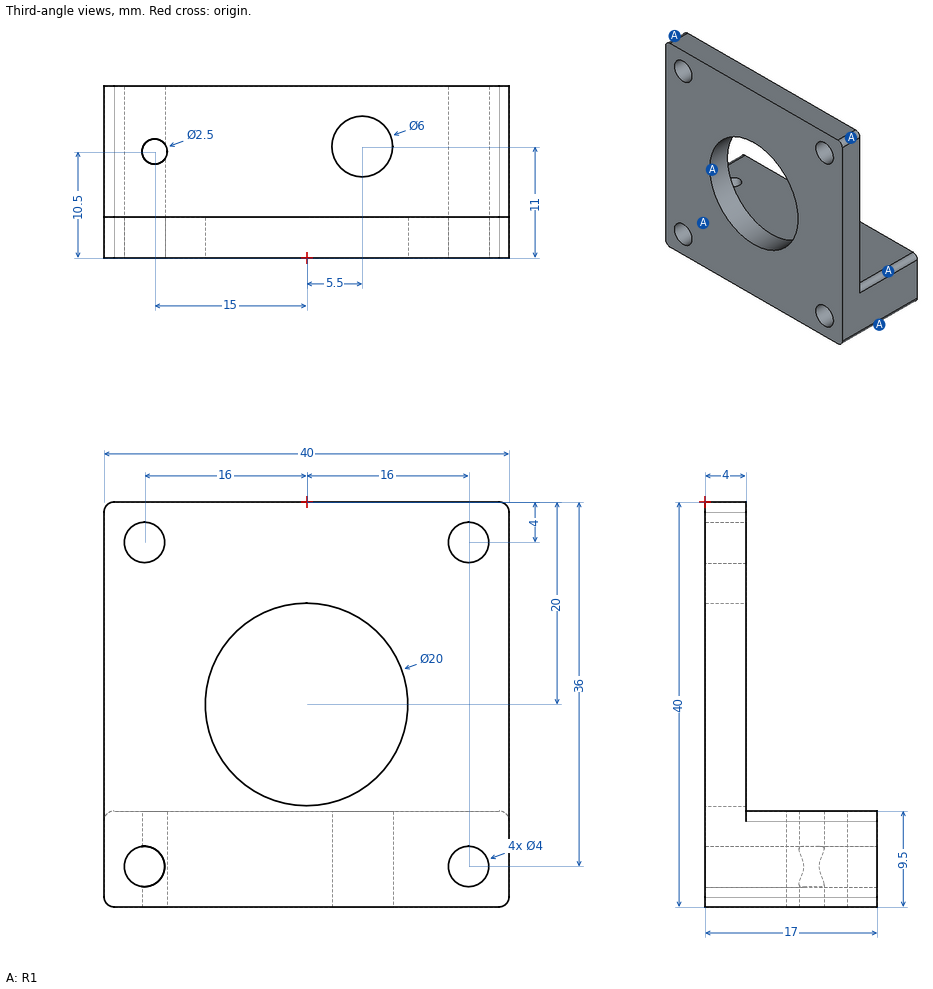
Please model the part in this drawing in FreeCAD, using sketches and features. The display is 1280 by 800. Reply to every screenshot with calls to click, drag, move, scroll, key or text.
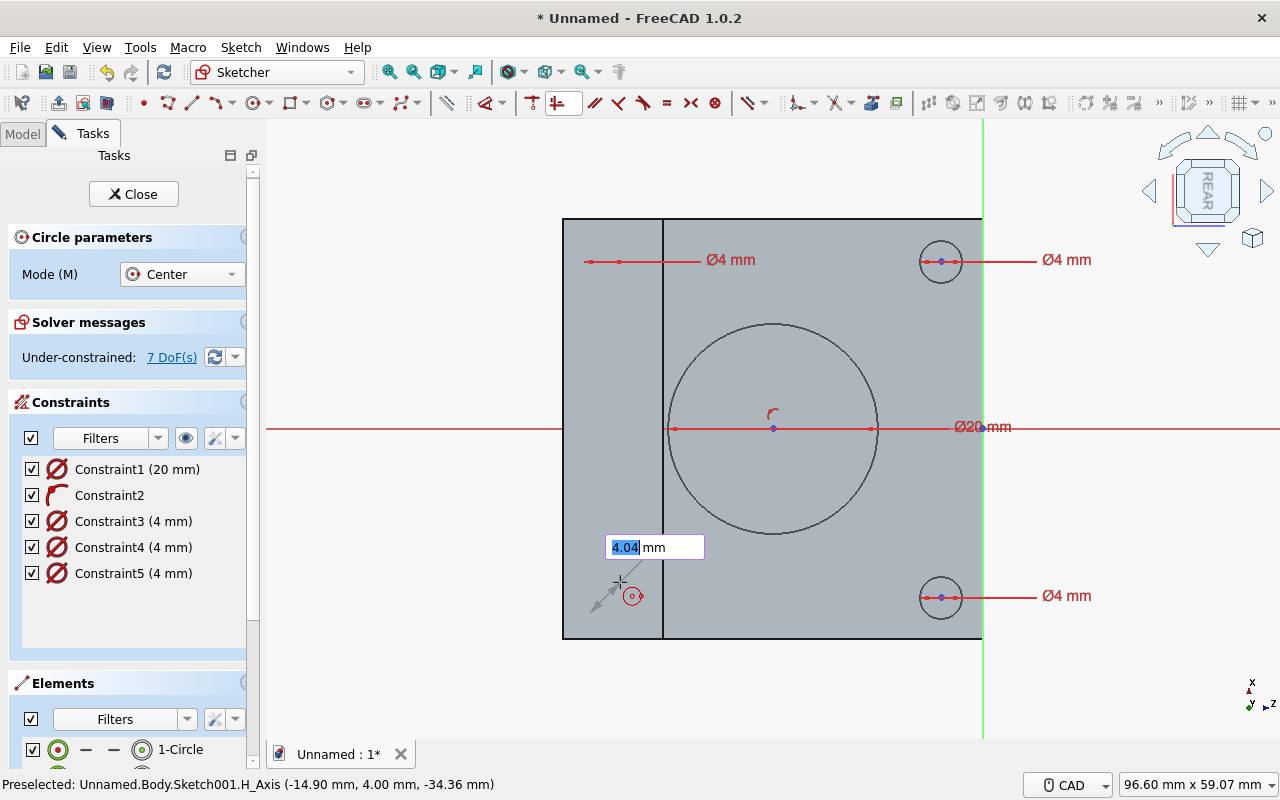
text(4)
key(Return)
key(Escape)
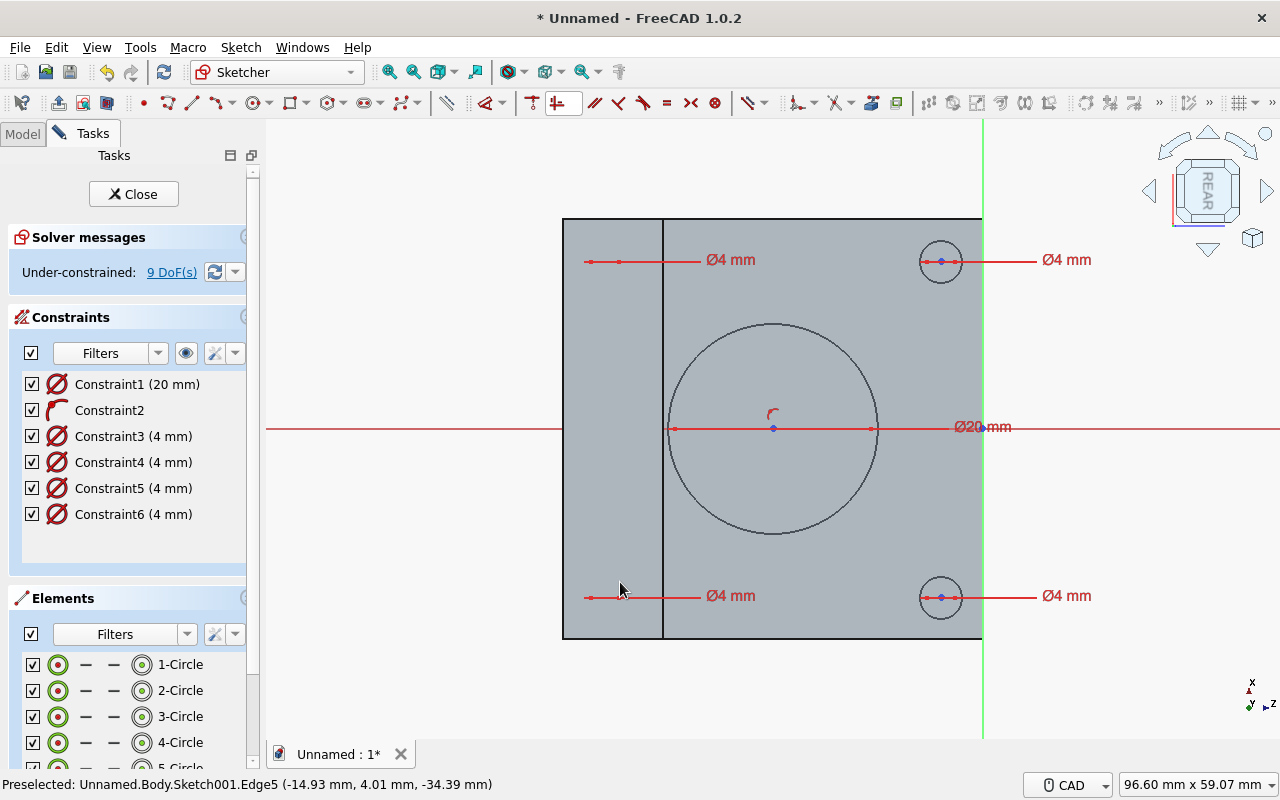
click(605, 262)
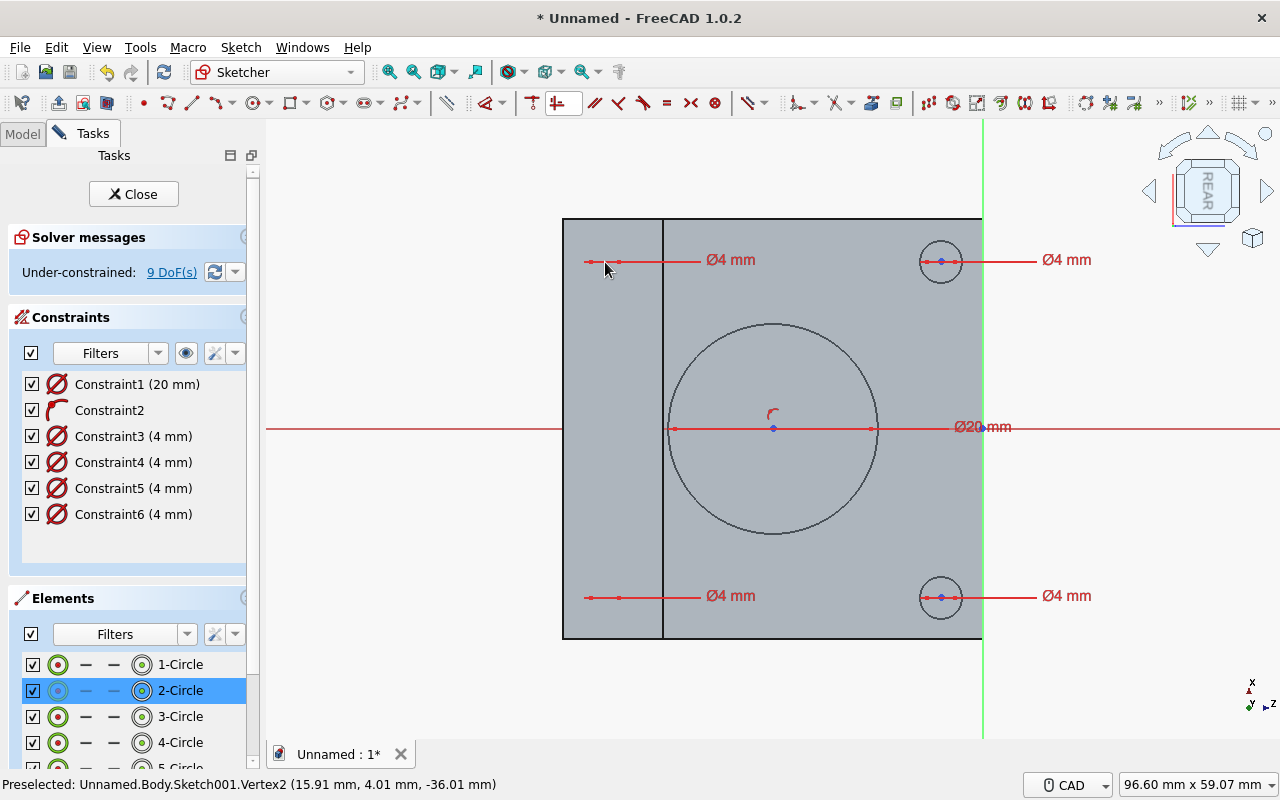
click(941, 262)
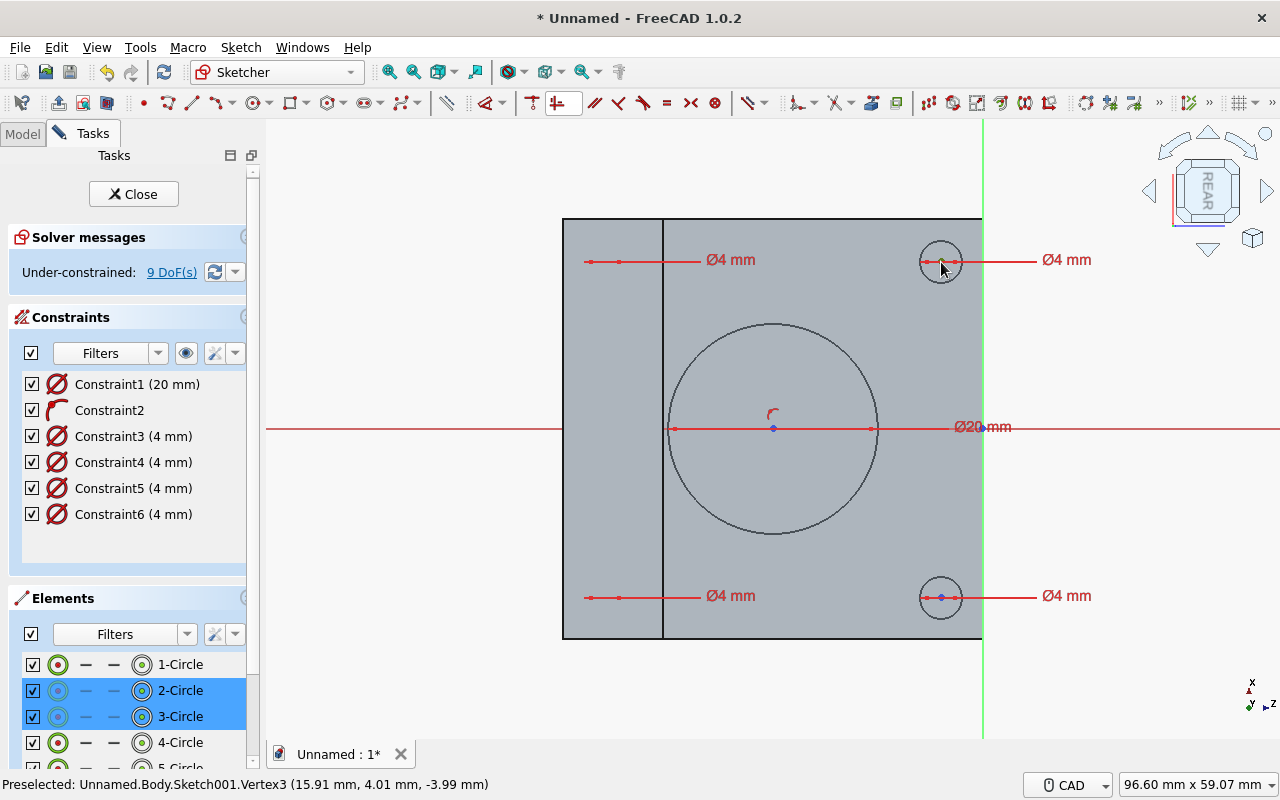
click(576, 104)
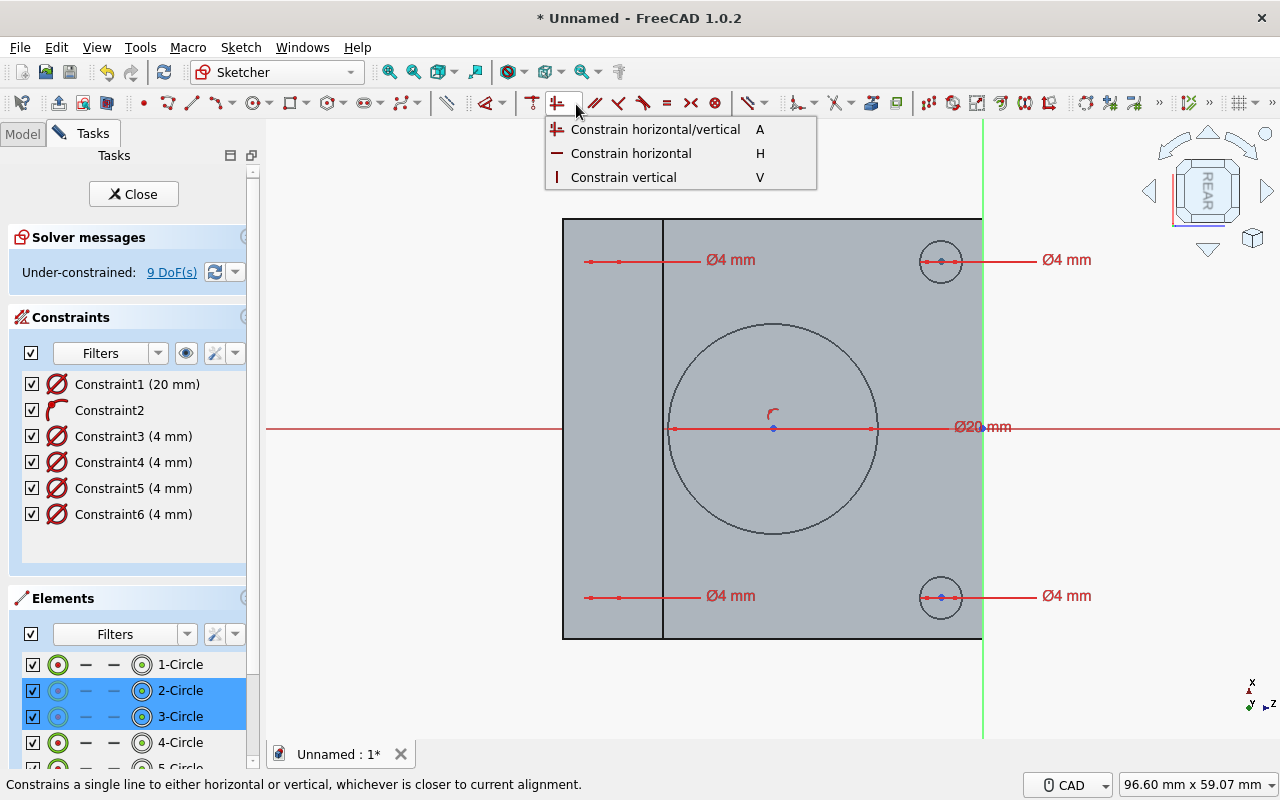
click(681, 153)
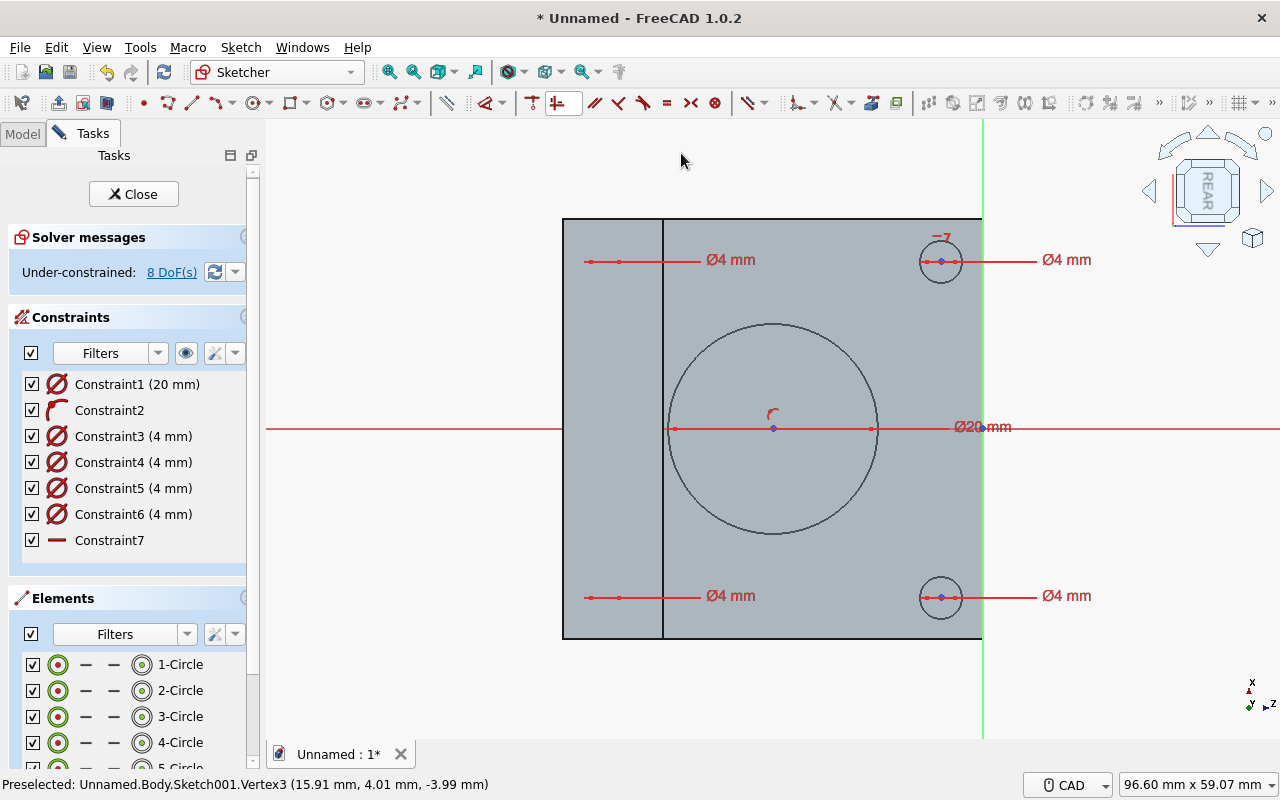
click(941, 262)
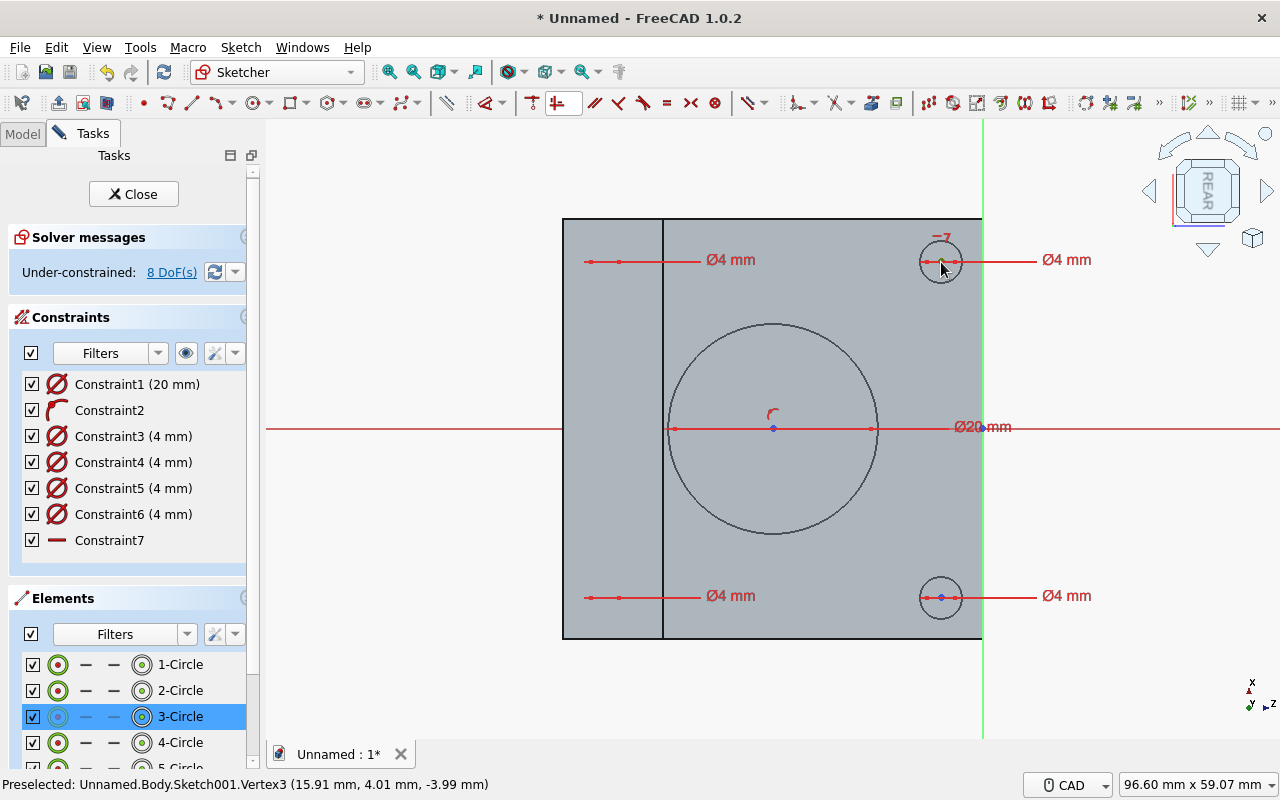
click(941, 598)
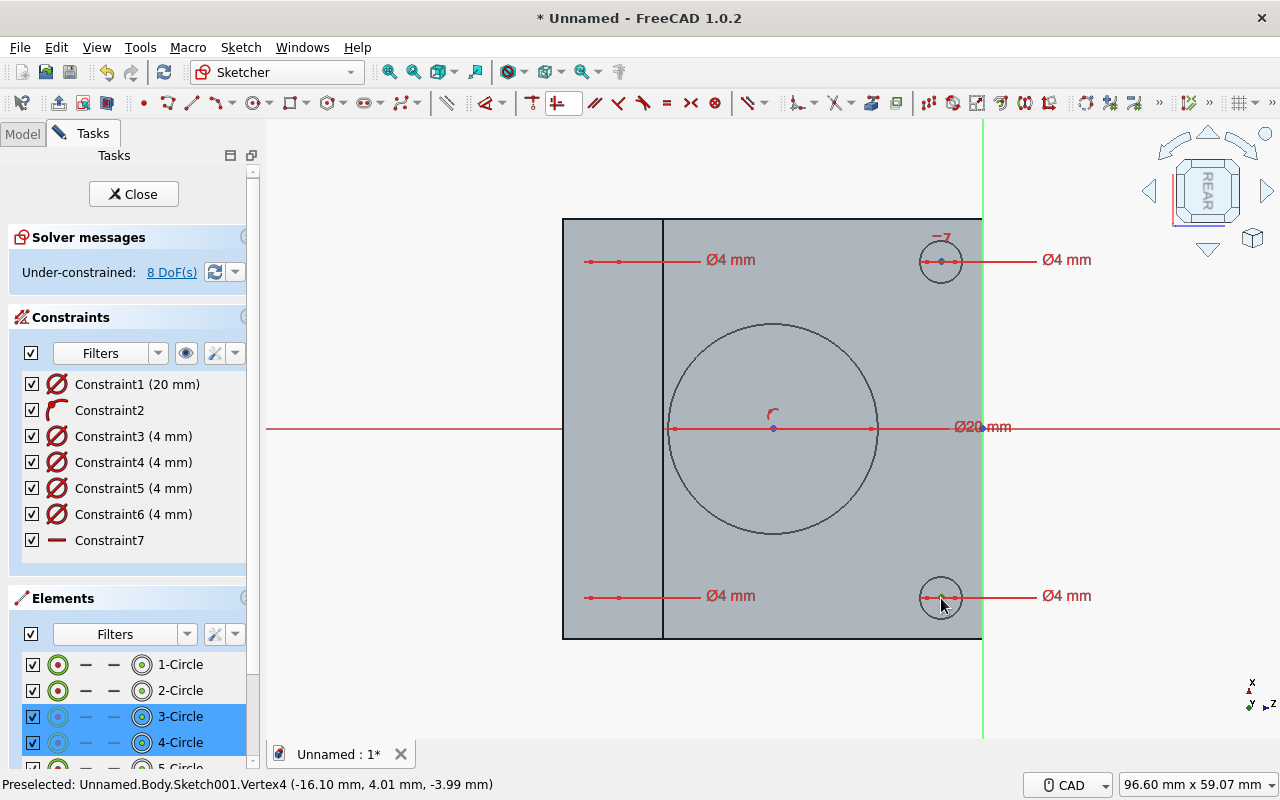
key(v)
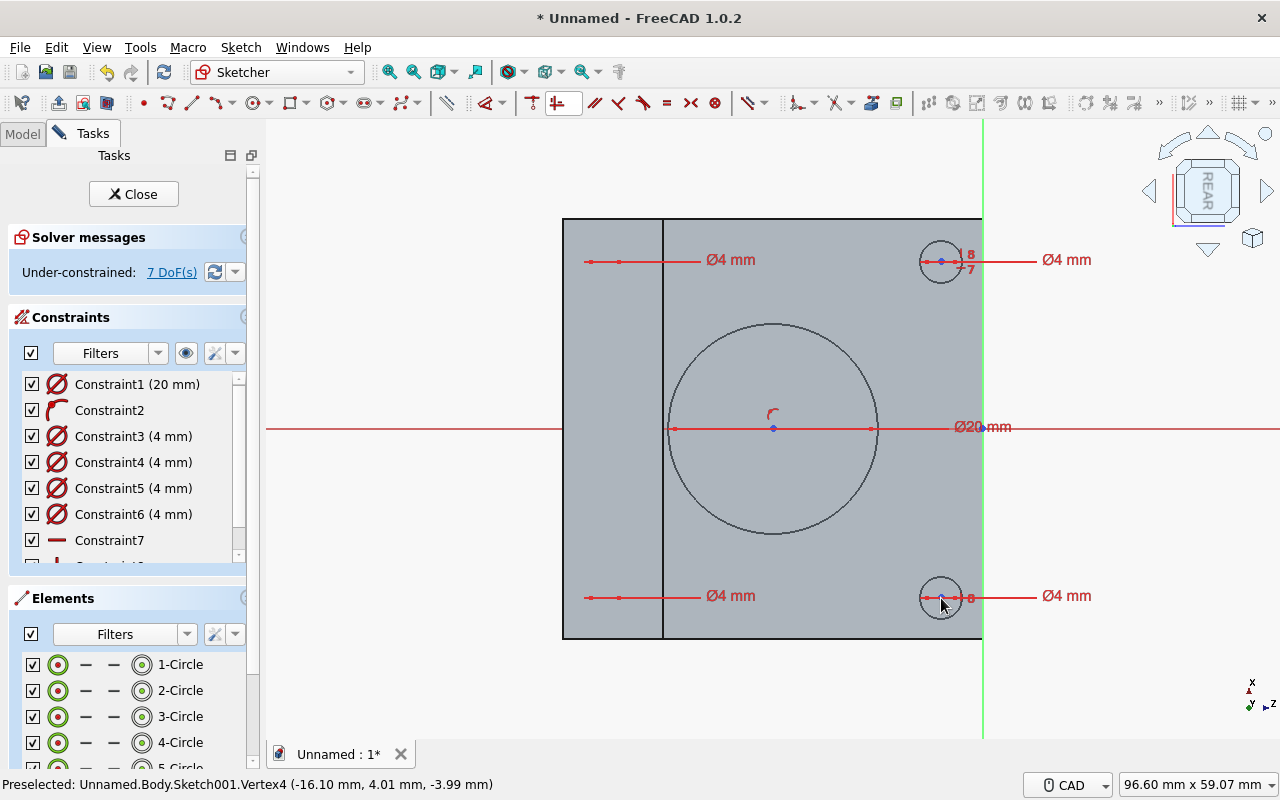
click(605, 262)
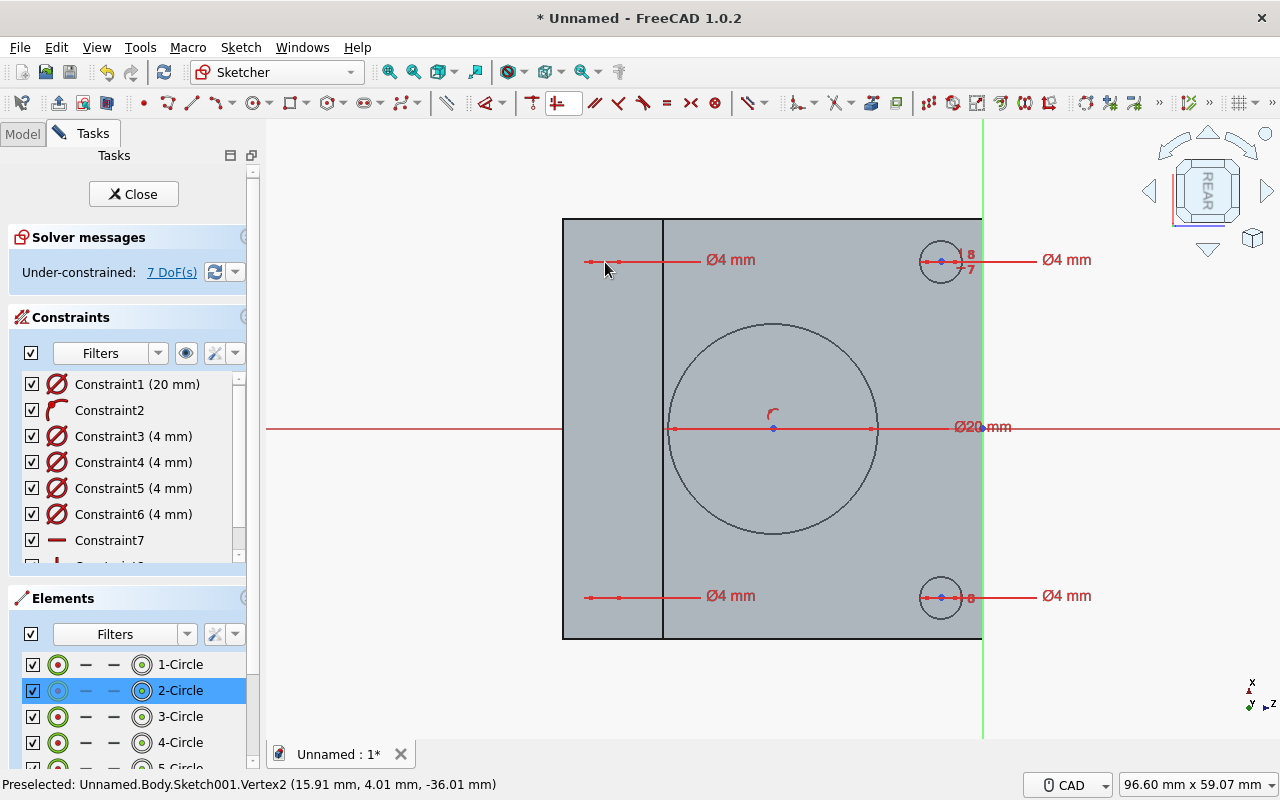
click(605, 598)